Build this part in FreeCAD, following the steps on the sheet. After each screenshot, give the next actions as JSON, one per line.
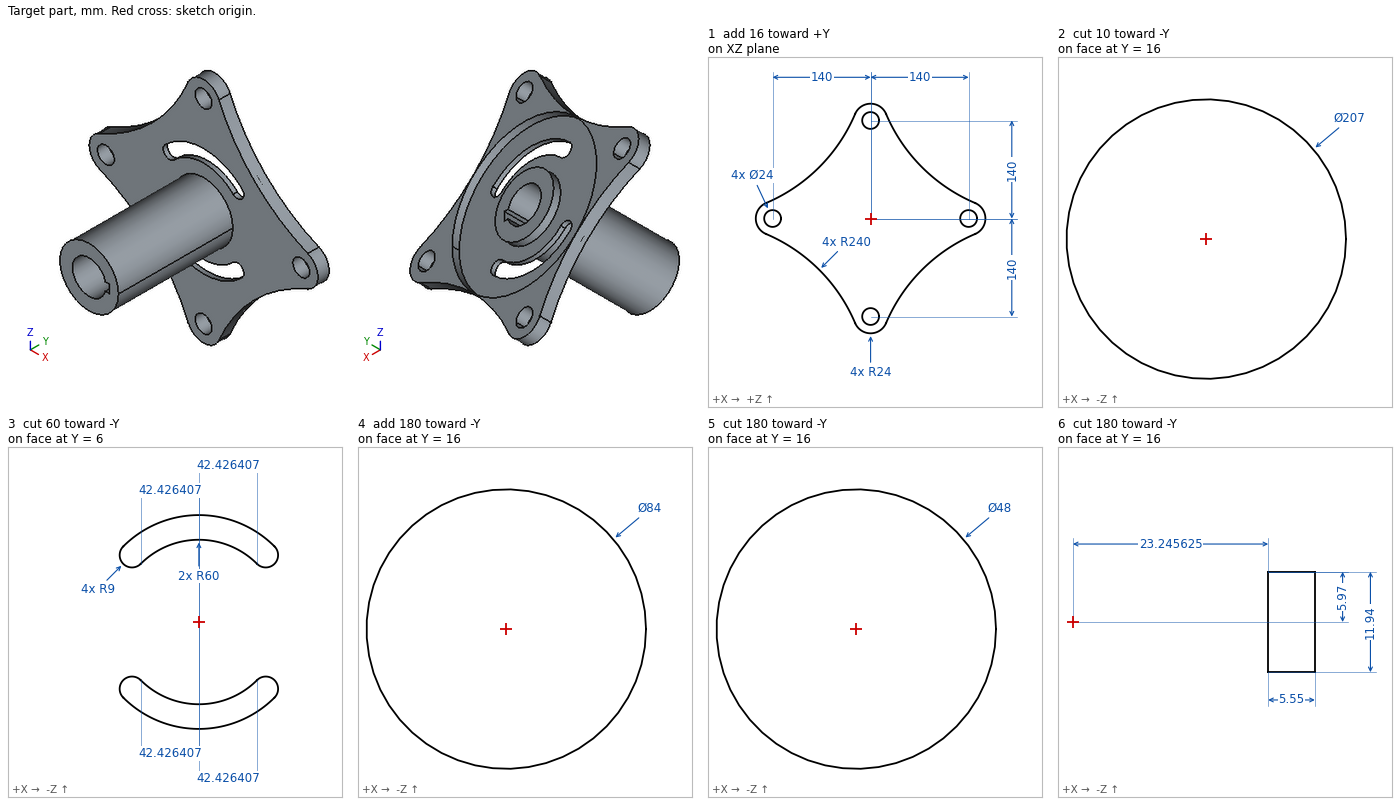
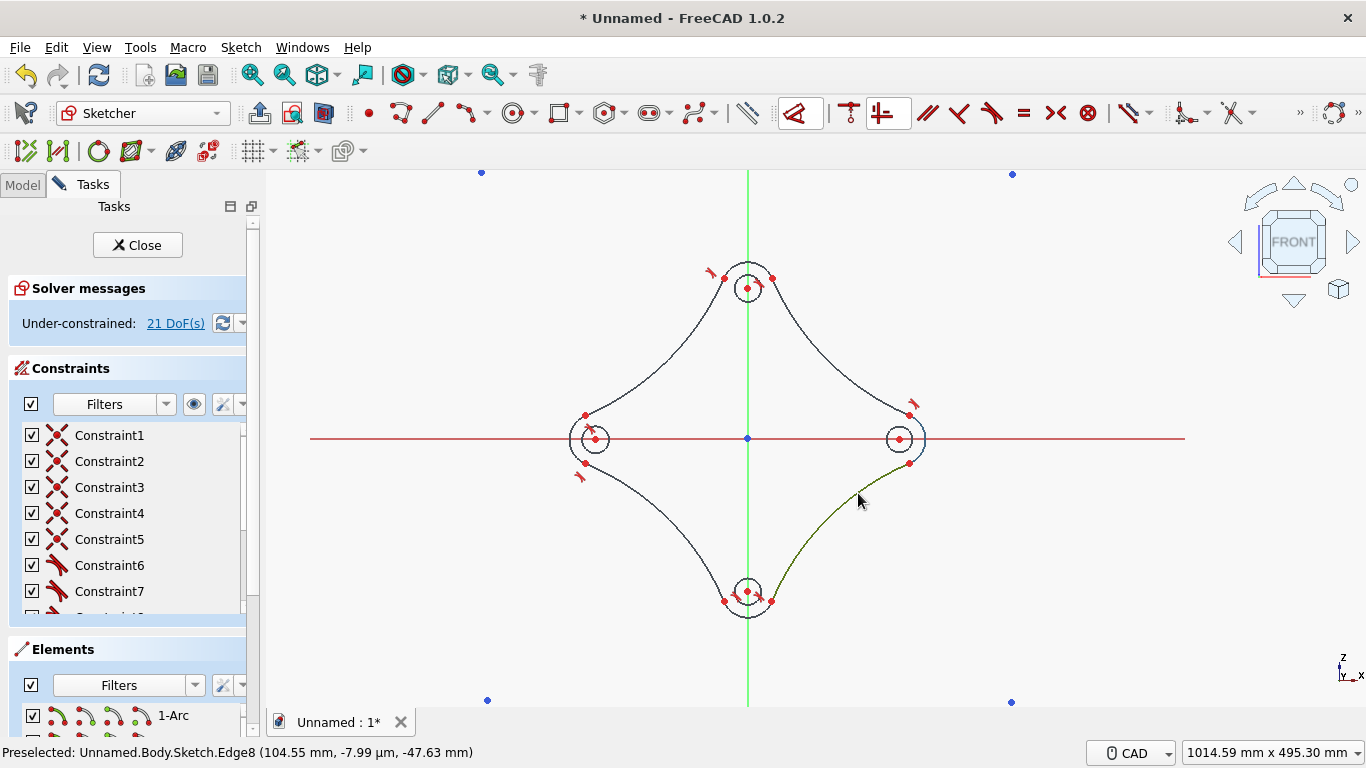
{"action": "left_click", "coordinate": [992, 114]}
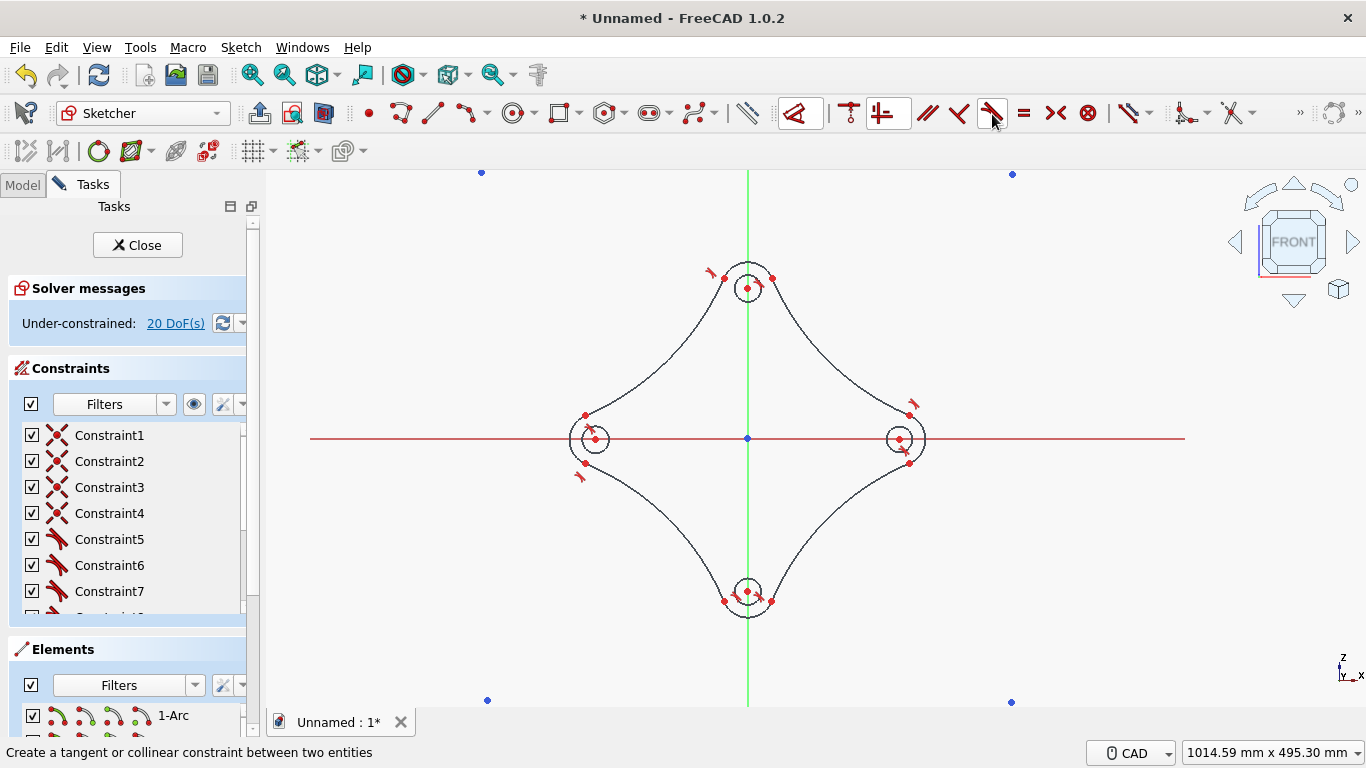
{"action": "left_click", "coordinate": [736, 615]}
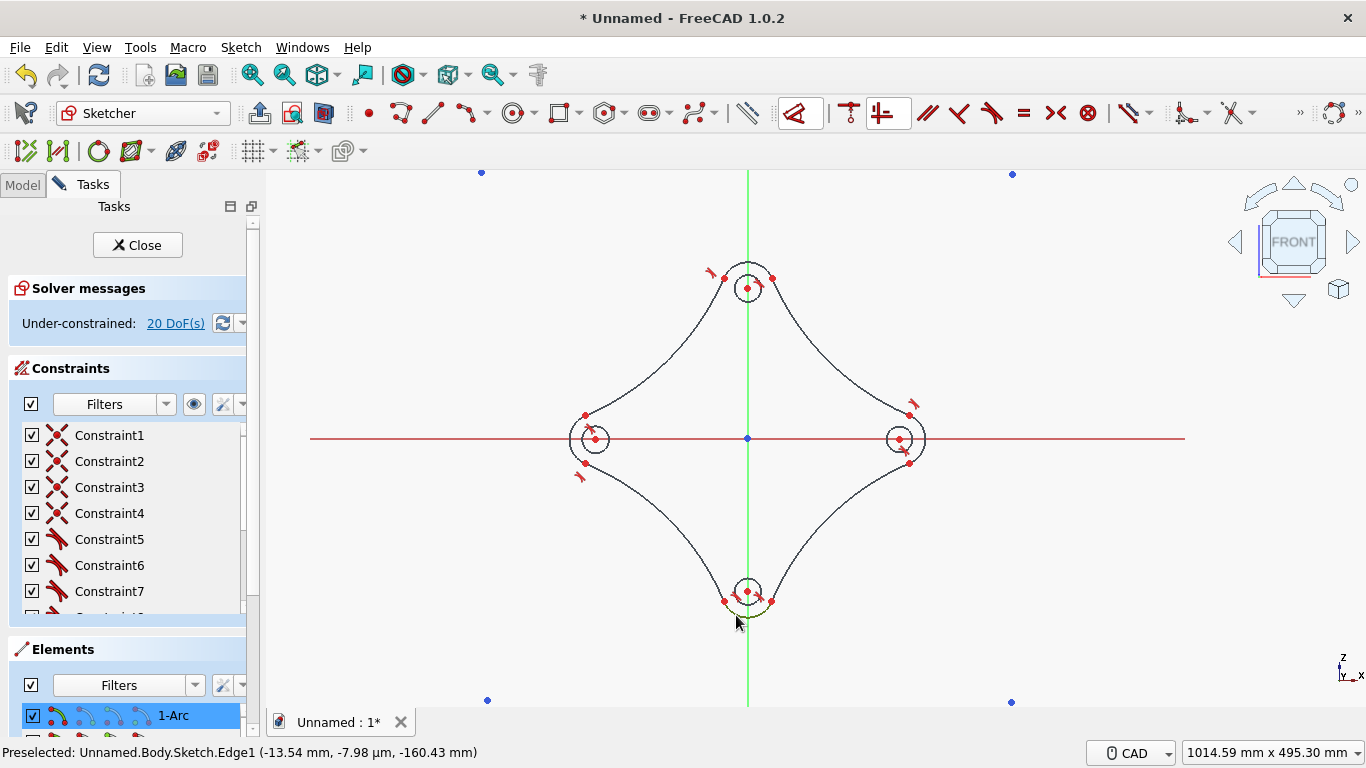
{"action": "scroll", "coordinate": [572, 428], "scroll_direction": "up", "scroll_amount": 2}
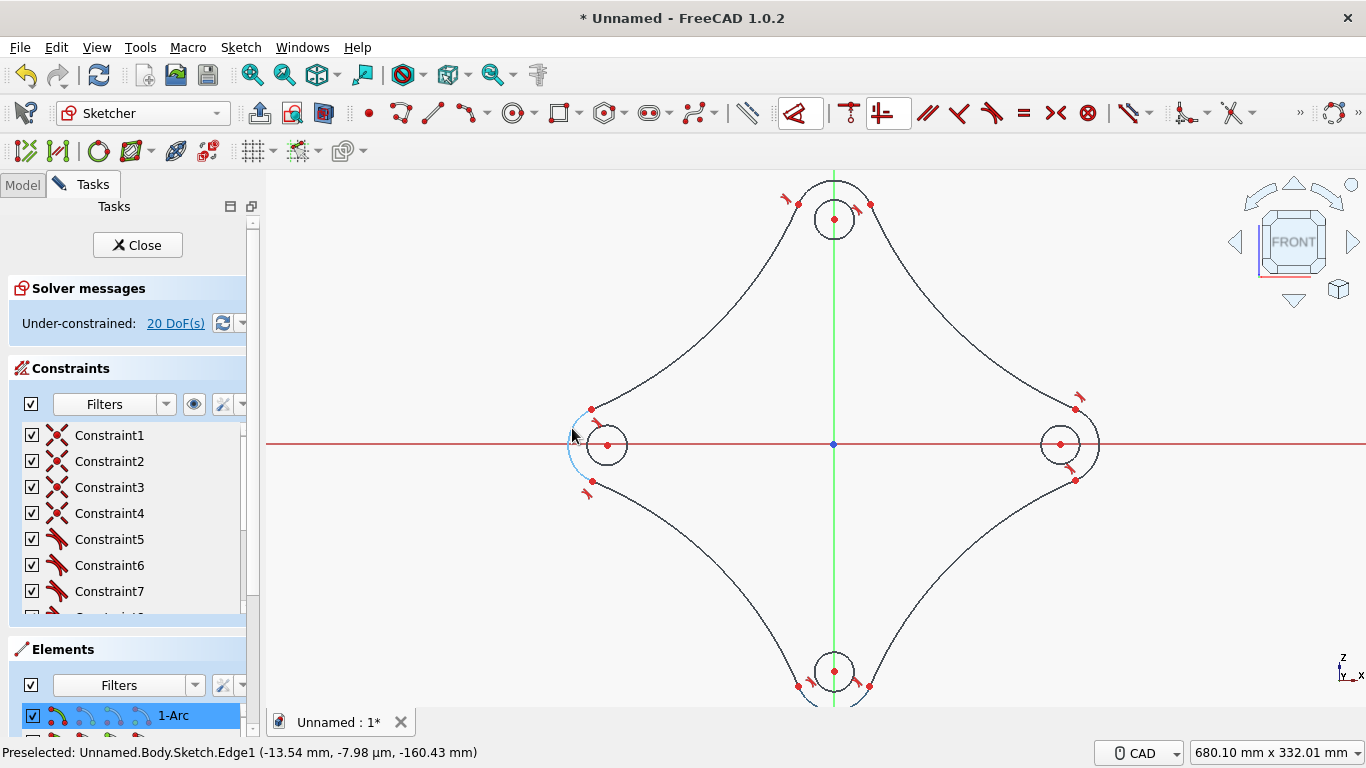
{"action": "left_click", "coordinate": [572, 428]}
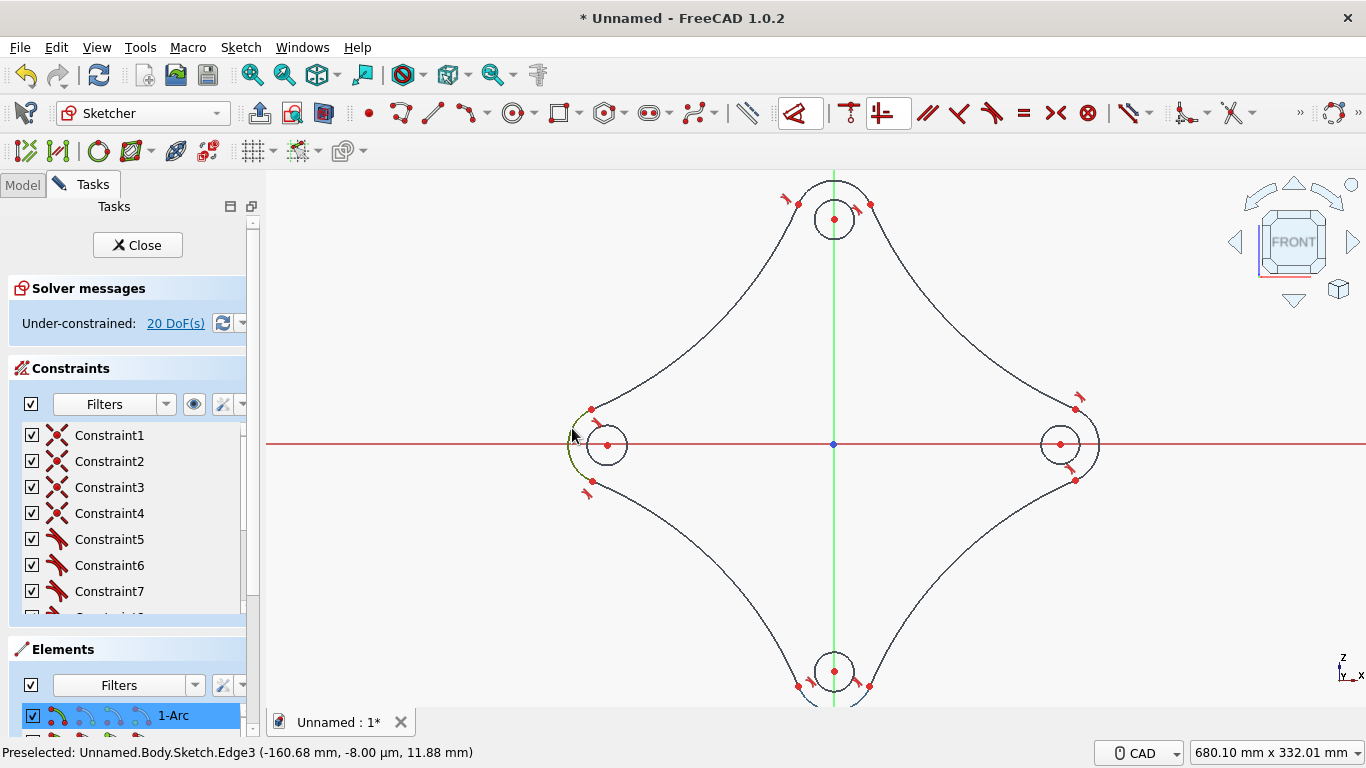
{"action": "scroll", "coordinate": [572, 427], "scroll_direction": "down", "scroll_amount": 2}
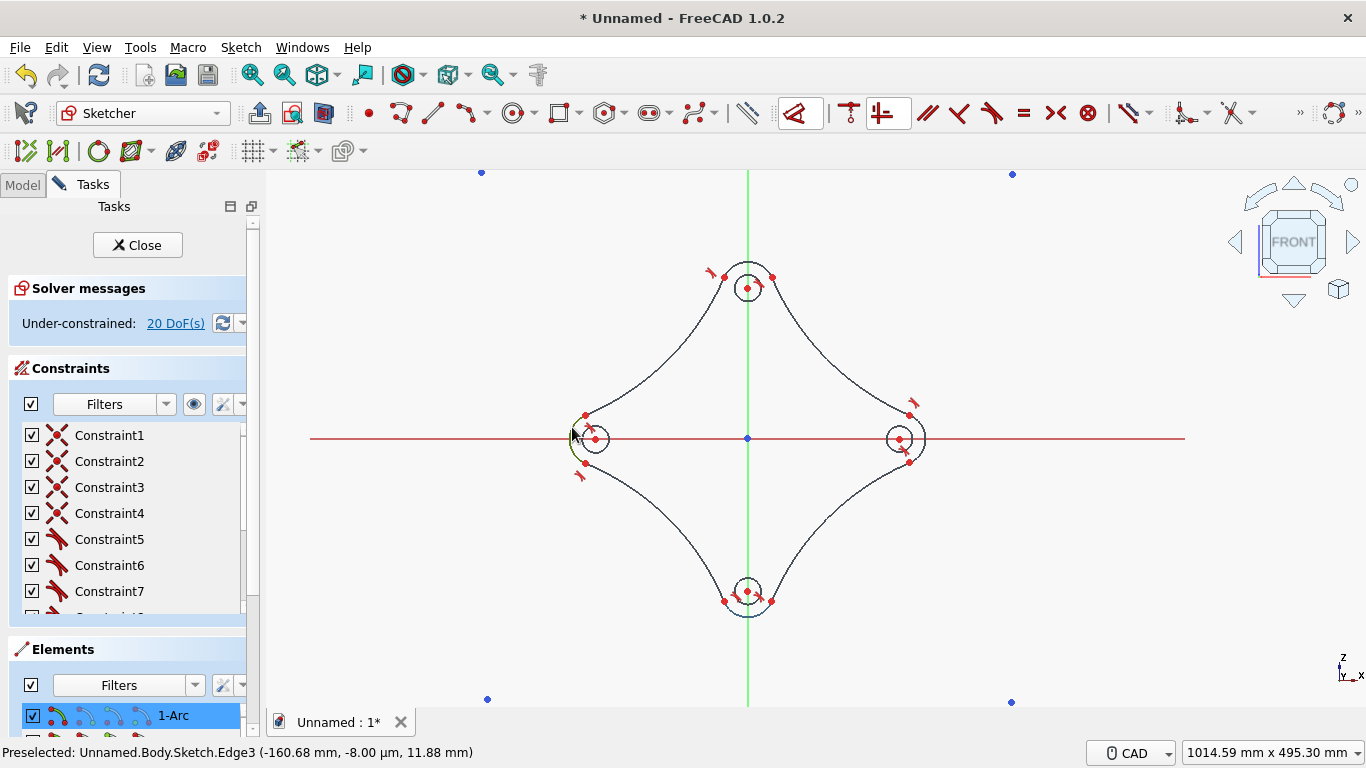
{"action": "left_click", "coordinate": [760, 265]}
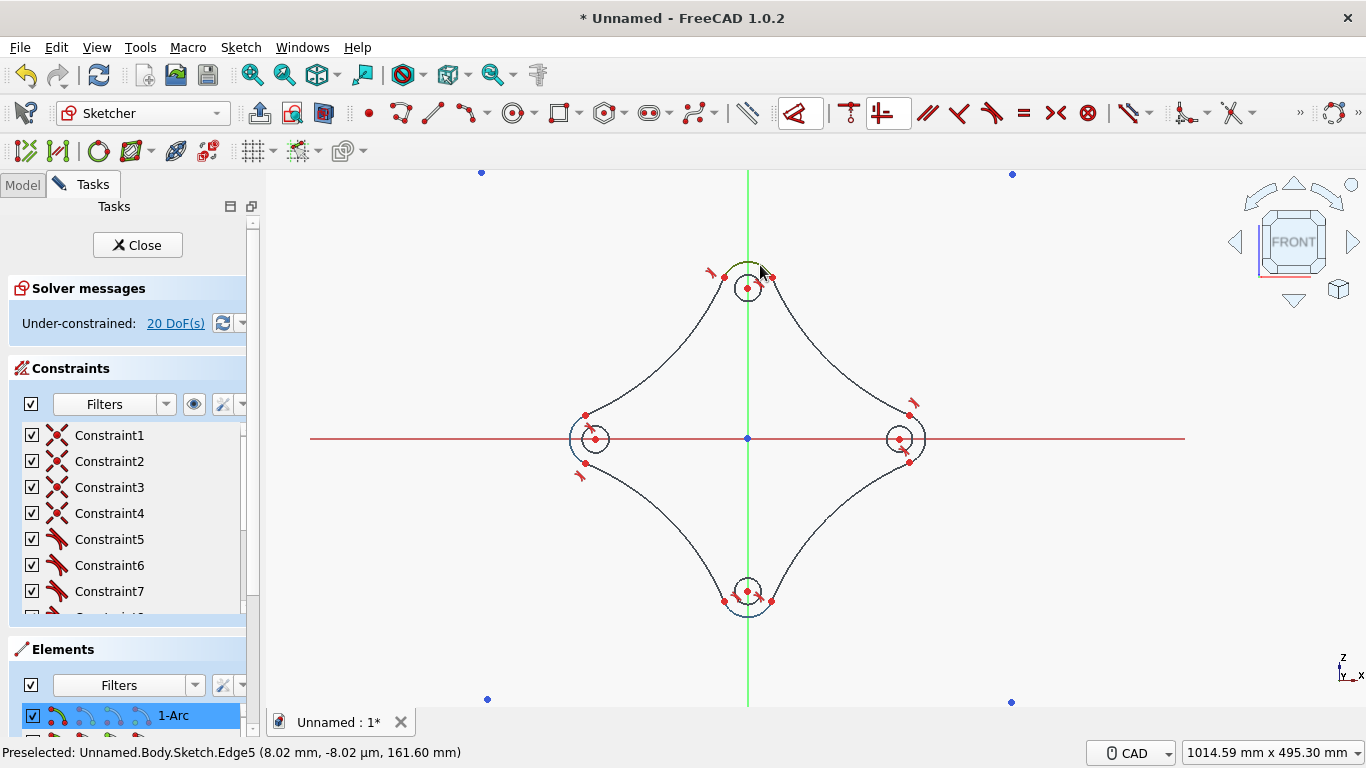
{"action": "left_click", "coordinate": [923, 451]}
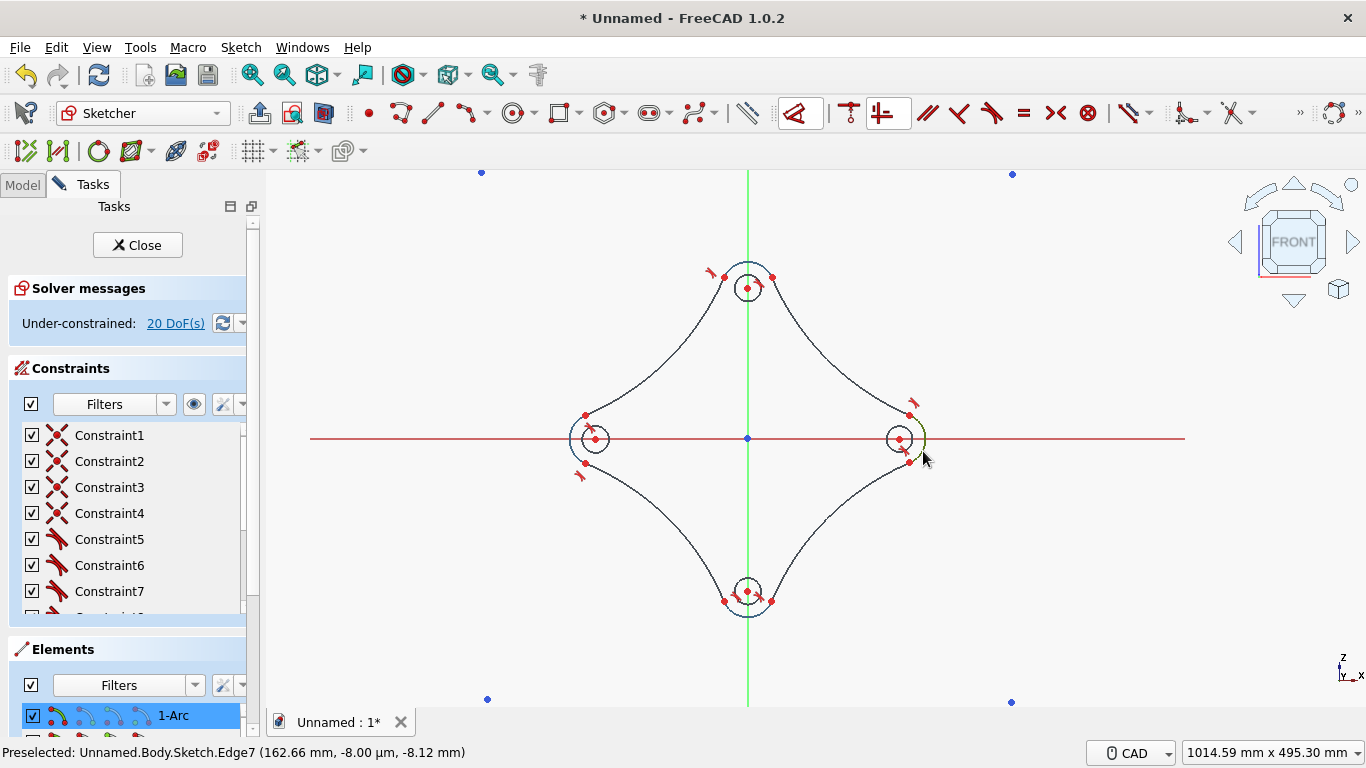
{"action": "left_click", "coordinate": [1024, 114]}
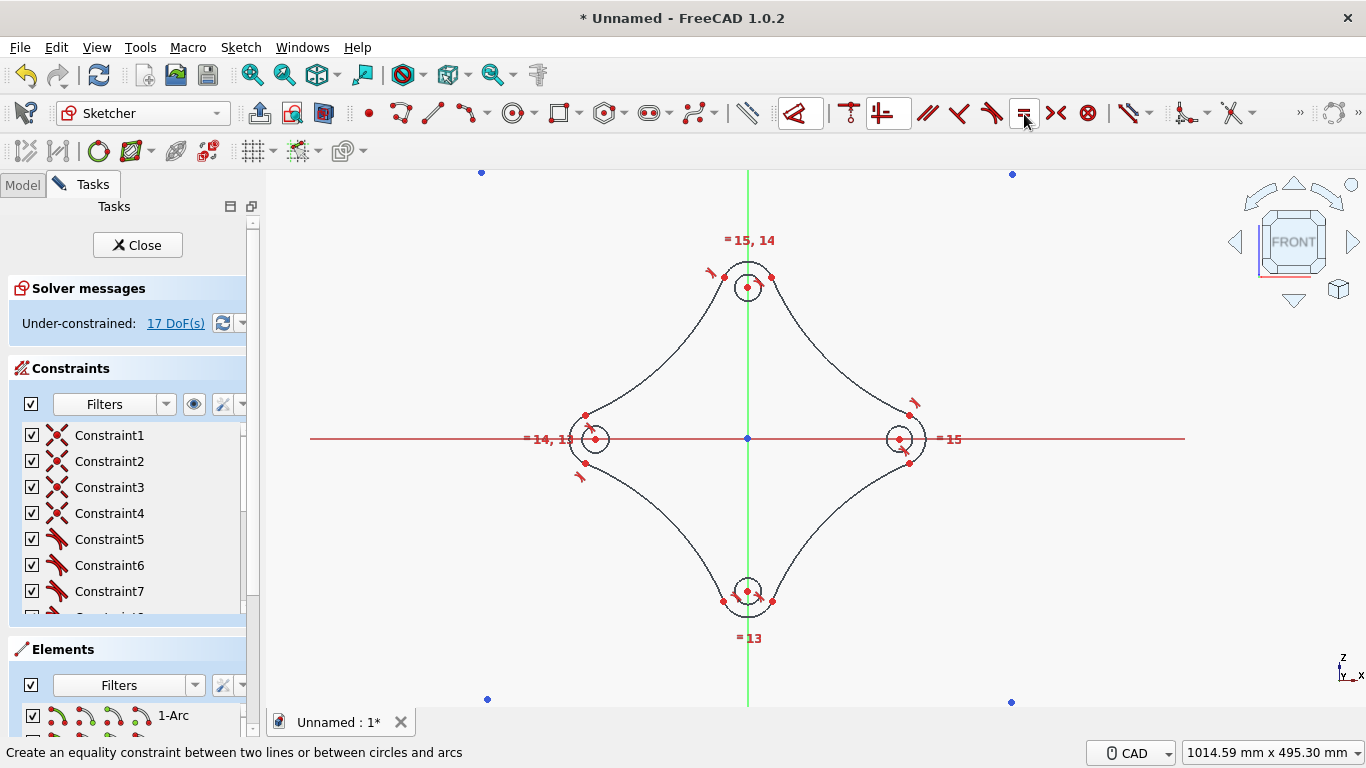
{"action": "left_click", "coordinate": [694, 549]}